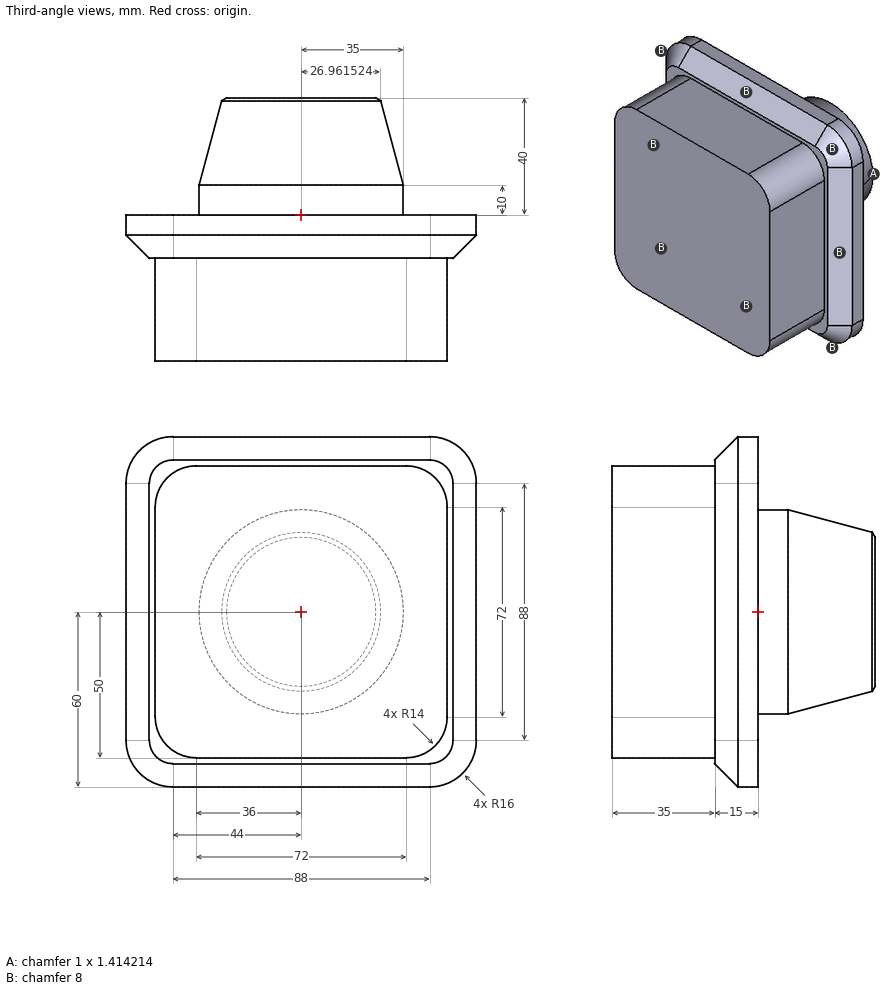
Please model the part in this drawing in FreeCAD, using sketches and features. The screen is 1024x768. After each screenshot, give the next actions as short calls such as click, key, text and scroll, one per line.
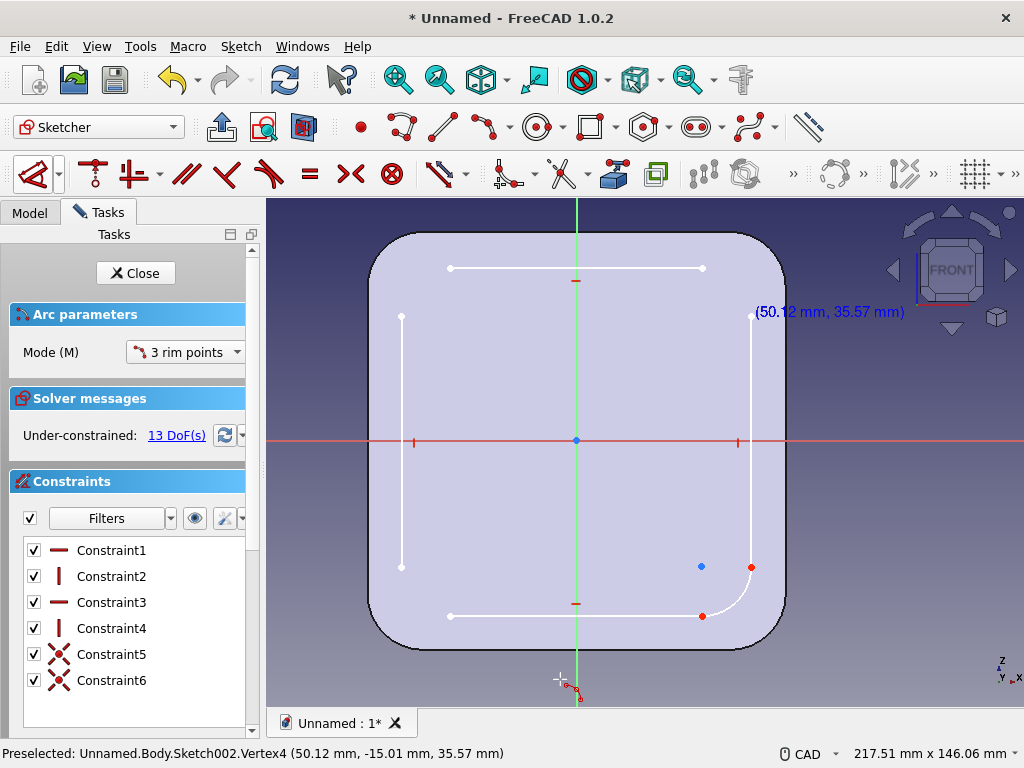
click(702, 268)
click(737, 281)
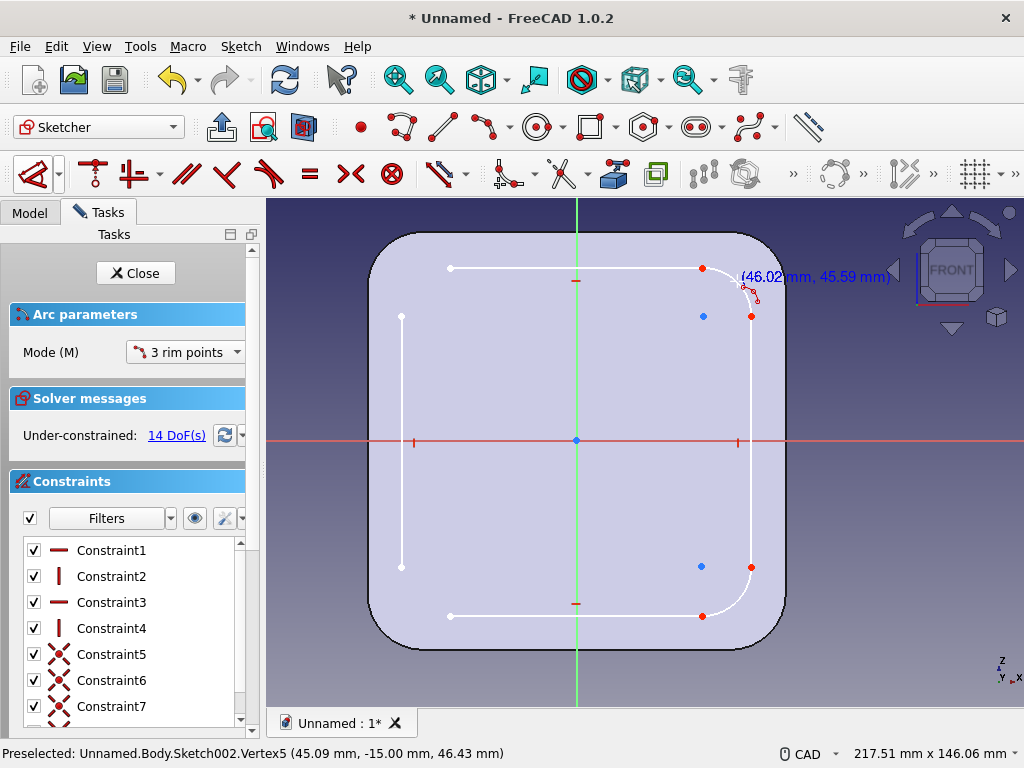
click(451, 268)
click(402, 317)
click(417, 281)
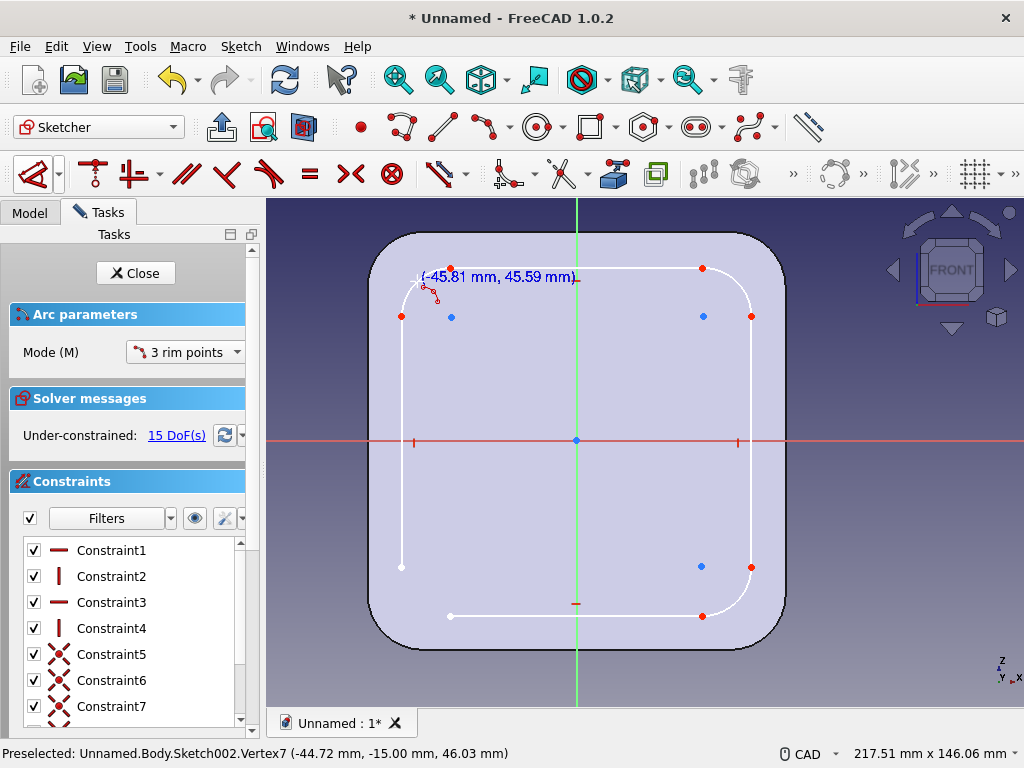
click(402, 567)
click(451, 616)
click(417, 601)
key(Escape)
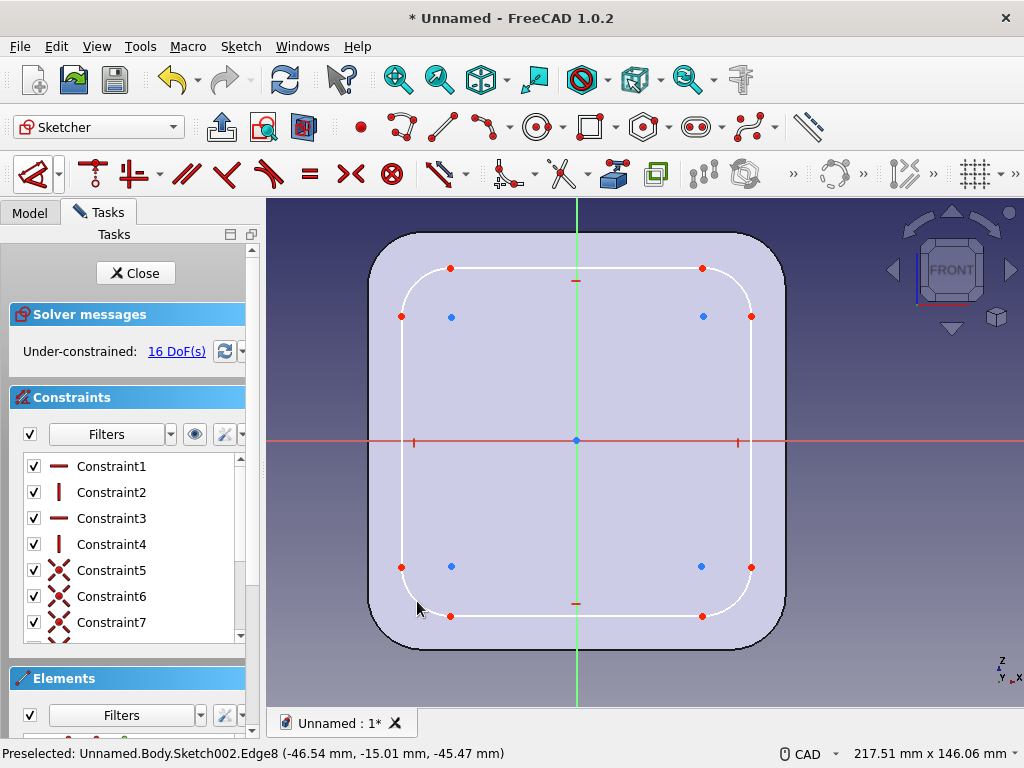
click(526, 616)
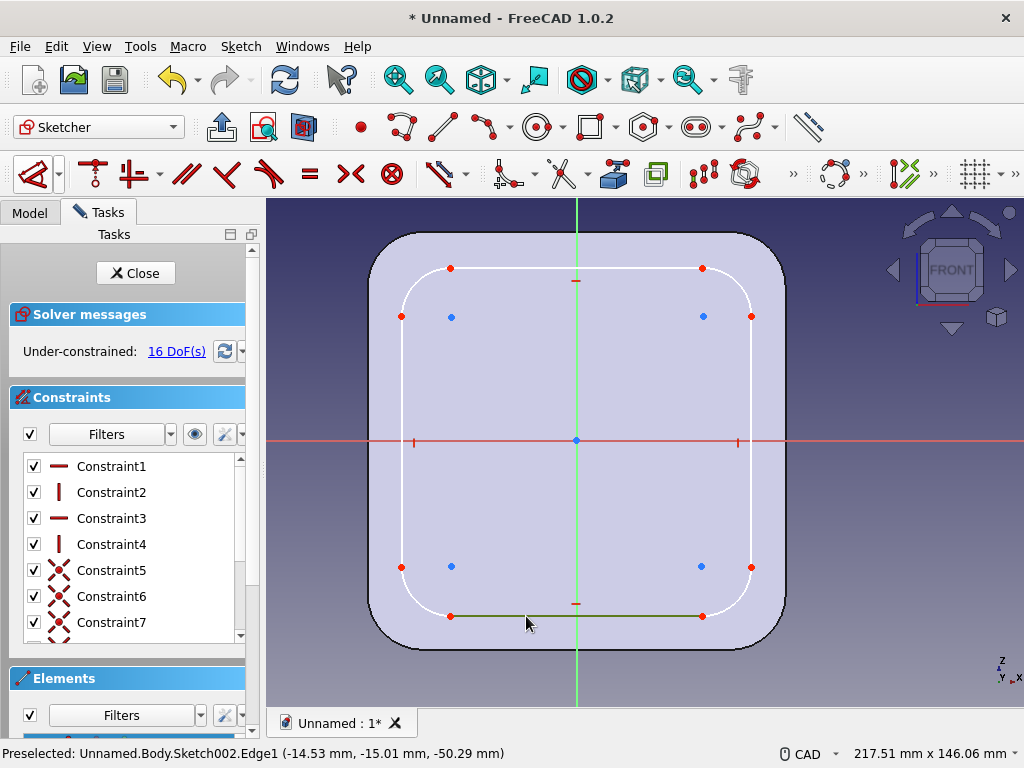
click(724, 611)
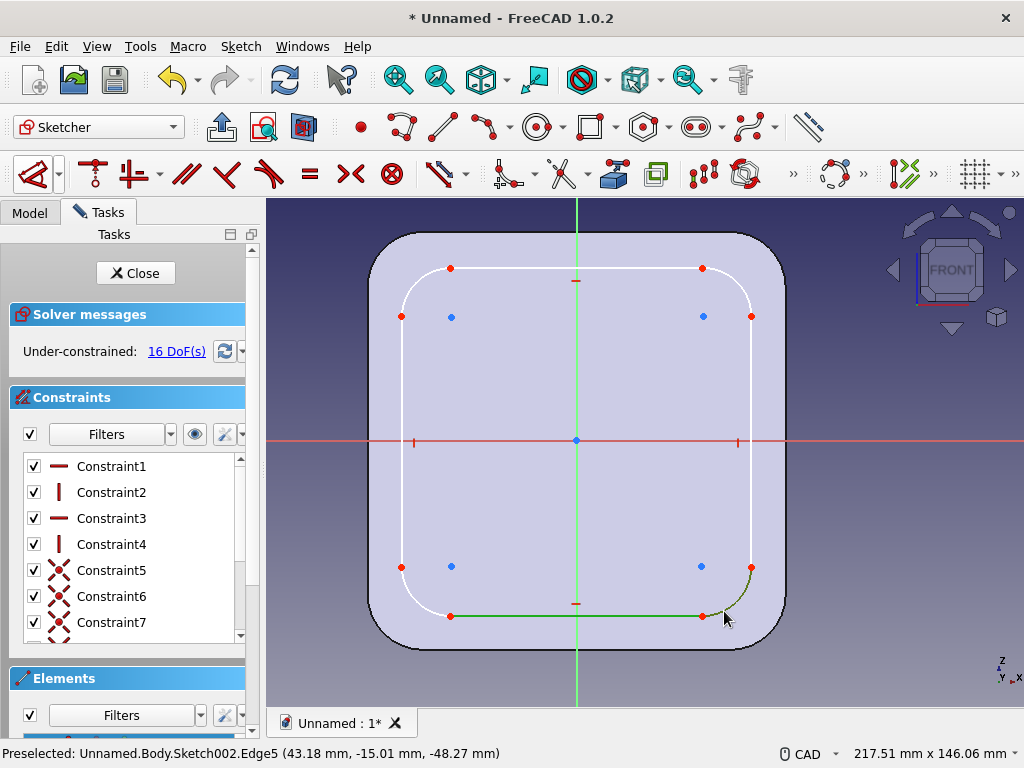
click(269, 174)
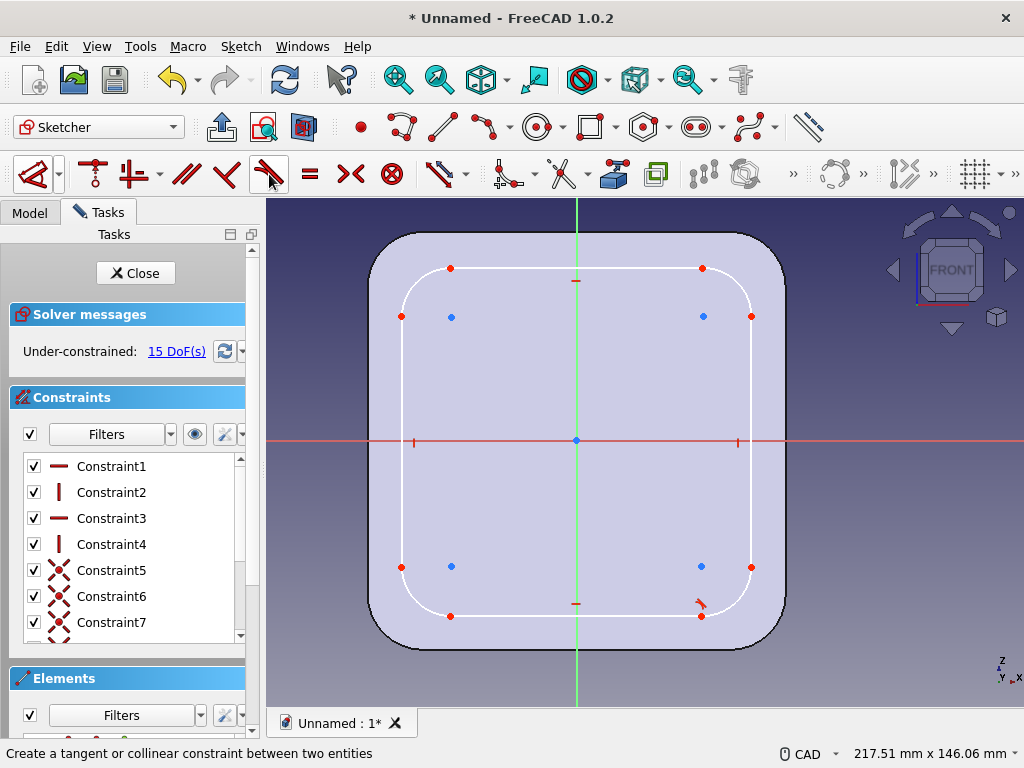
click(526, 616)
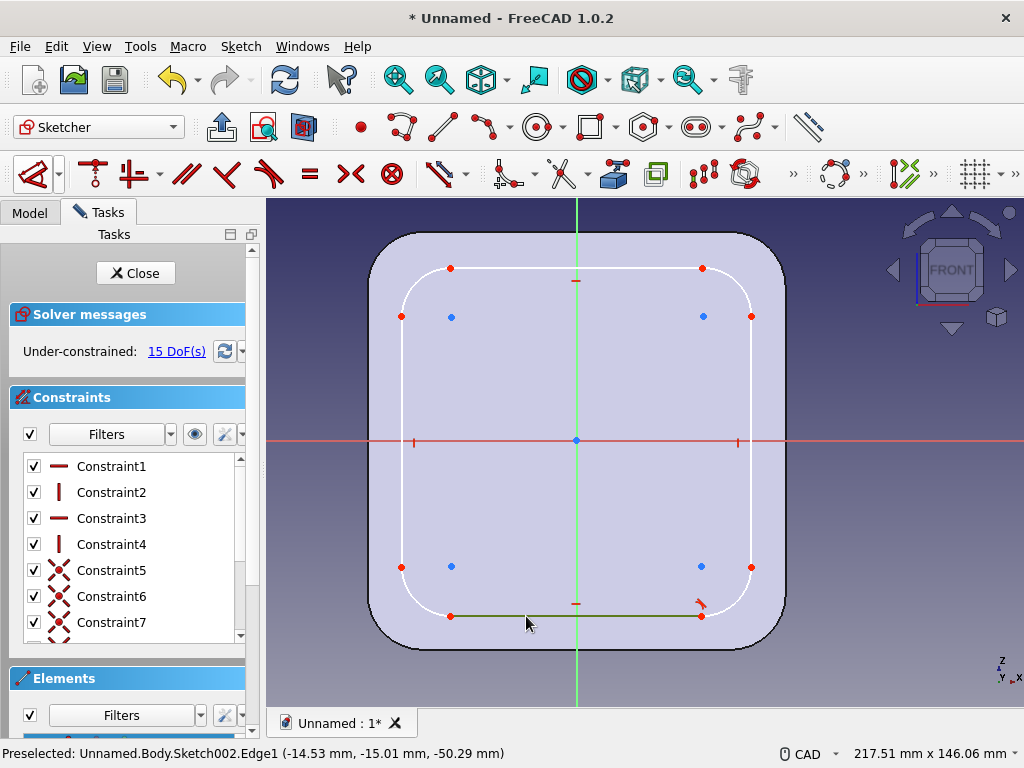
click(408, 589)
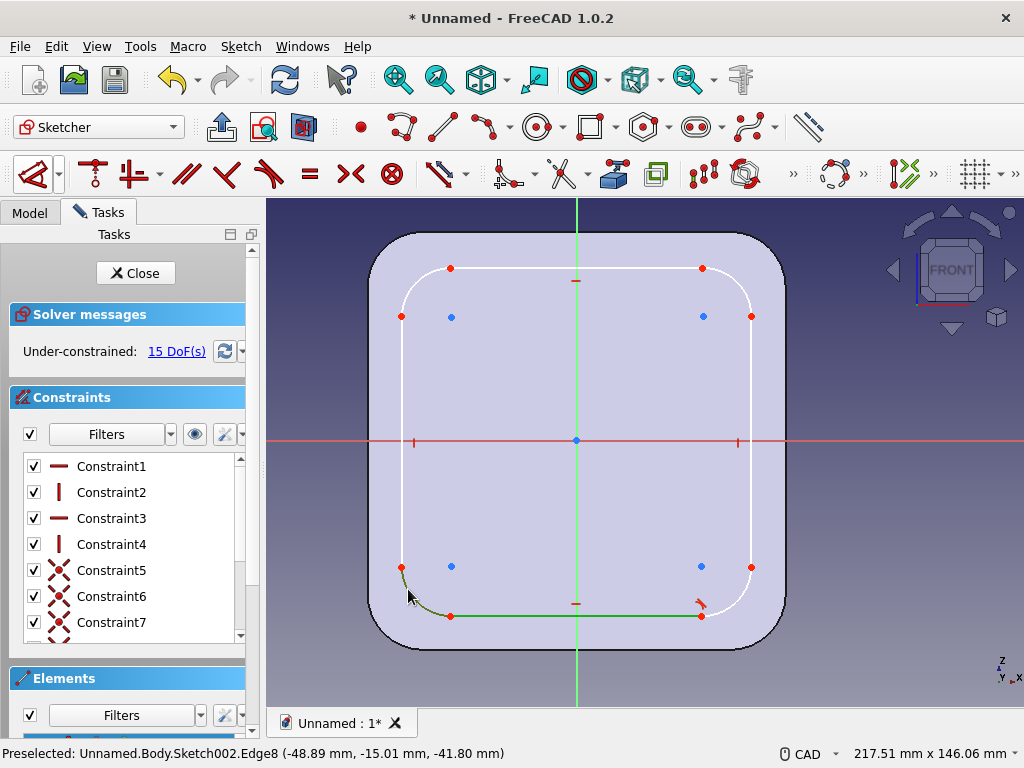
key(t)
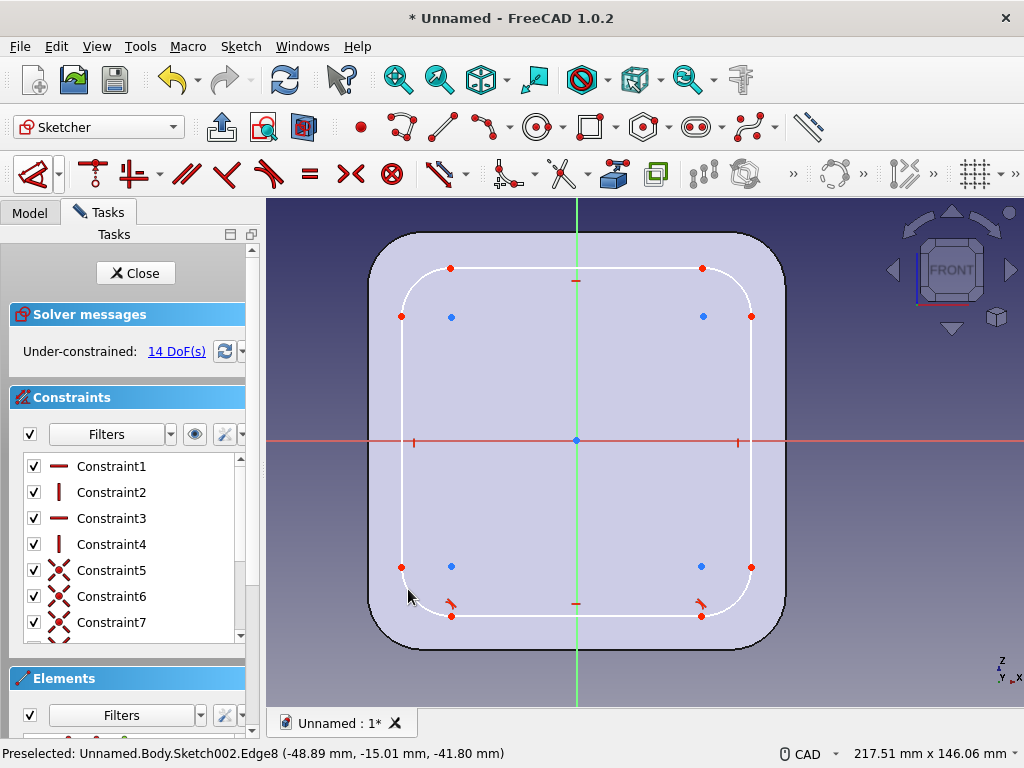
click(751, 492)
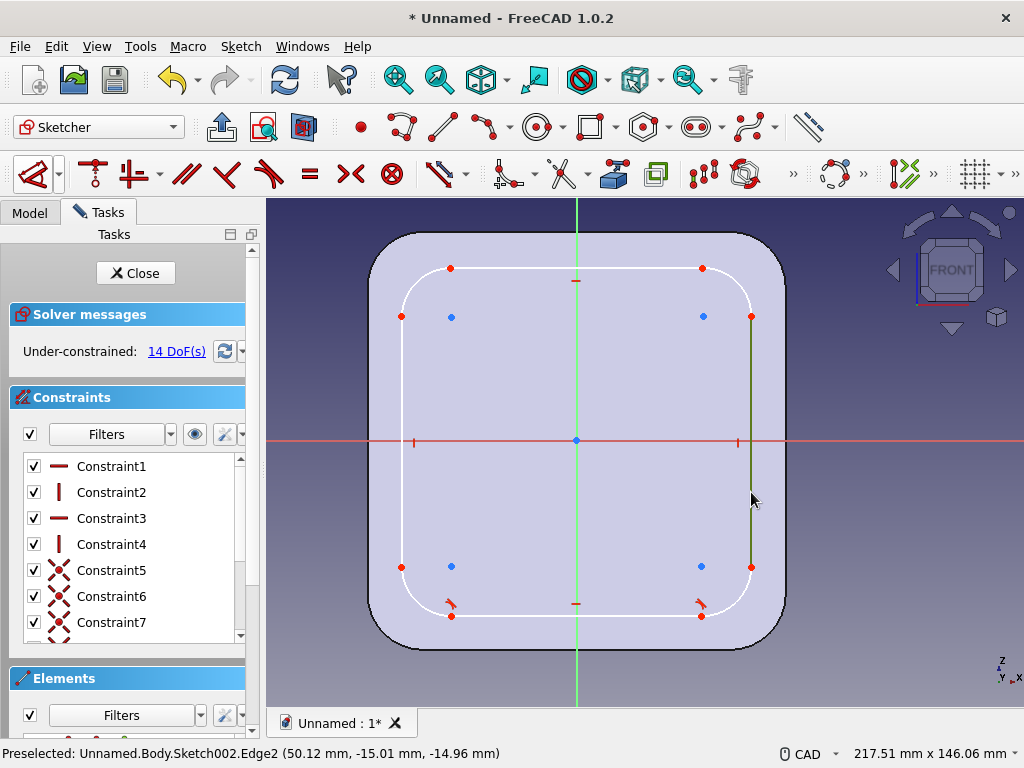
click(724, 611)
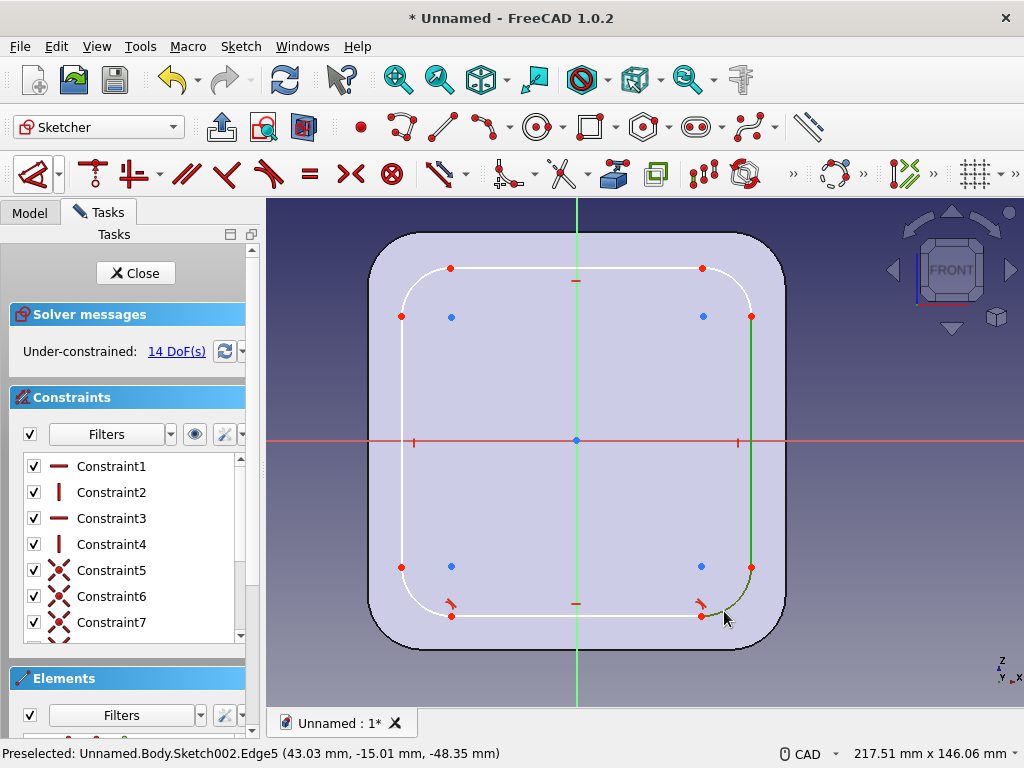
click(269, 174)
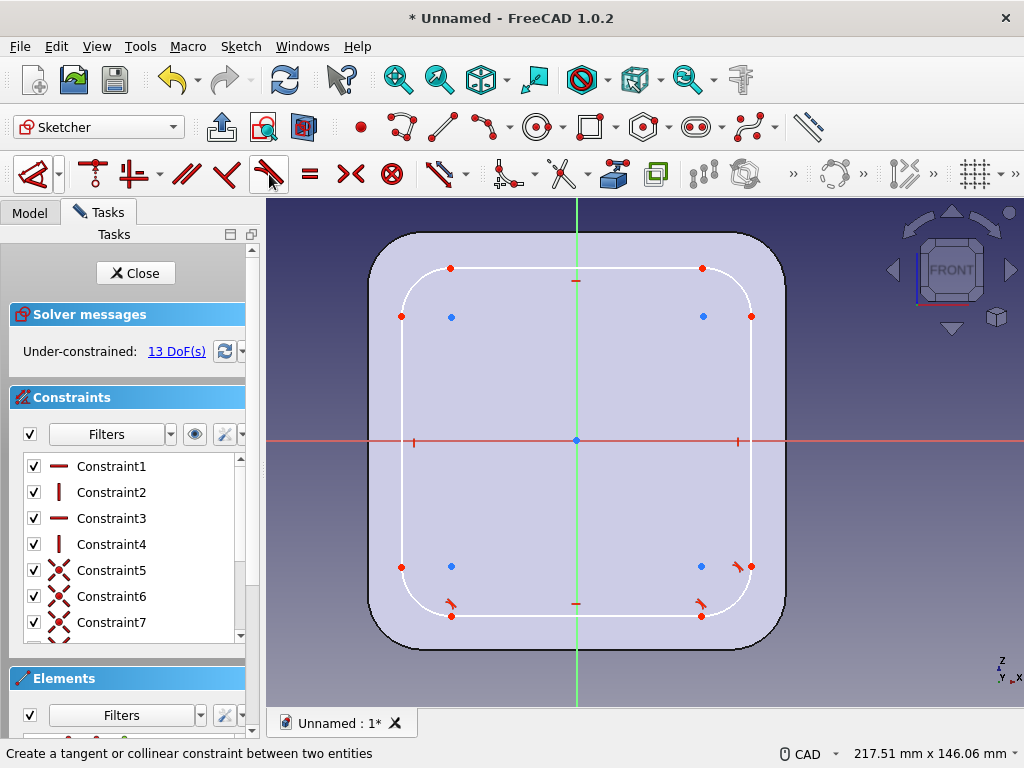
click(751, 492)